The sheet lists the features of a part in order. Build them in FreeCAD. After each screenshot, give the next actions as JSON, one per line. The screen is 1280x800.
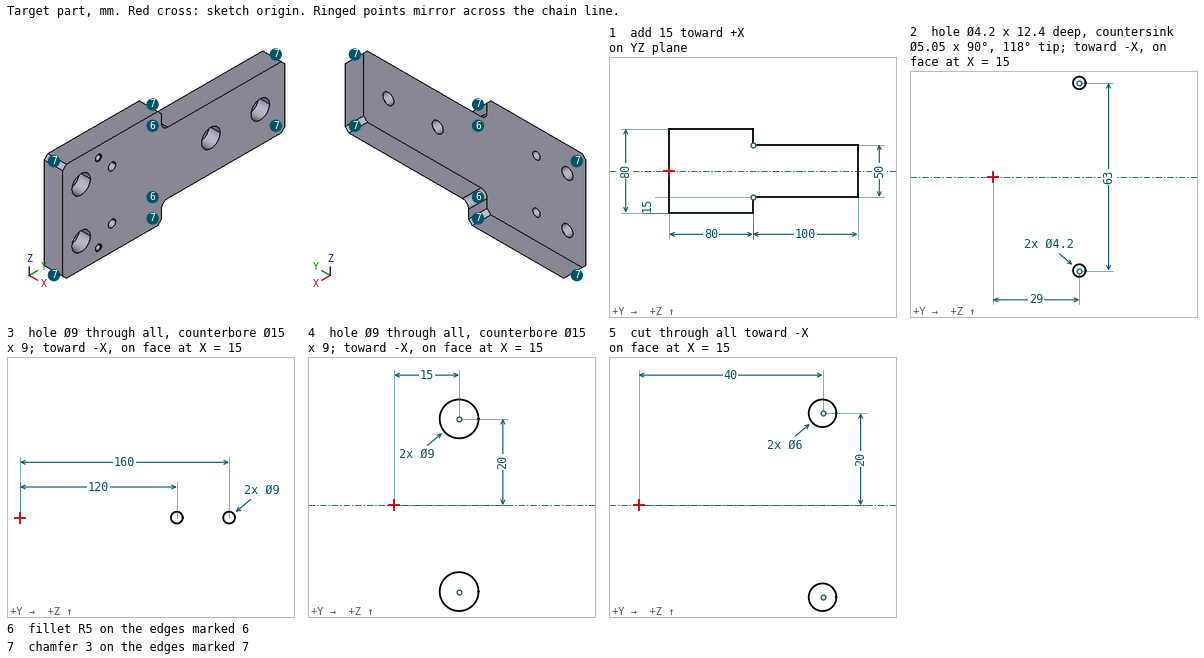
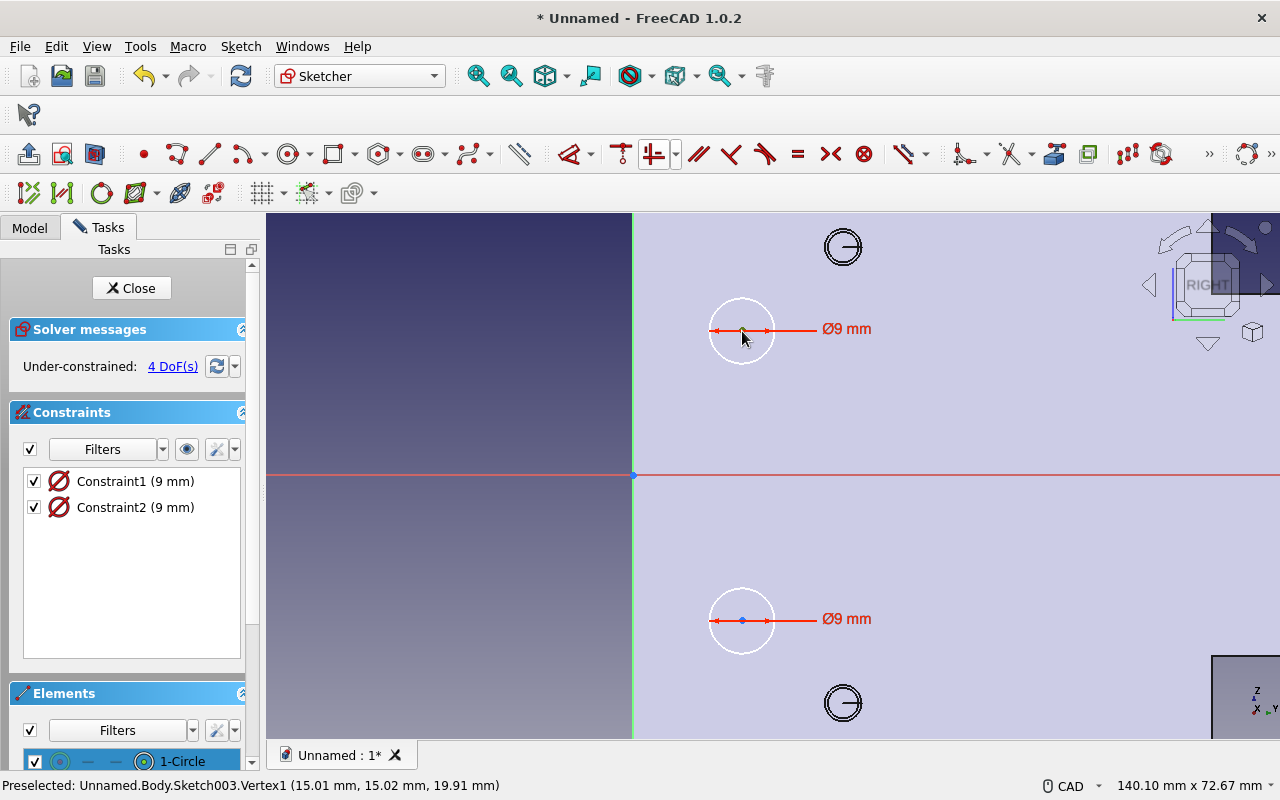
{"action": "left_click", "coordinate": [742, 621]}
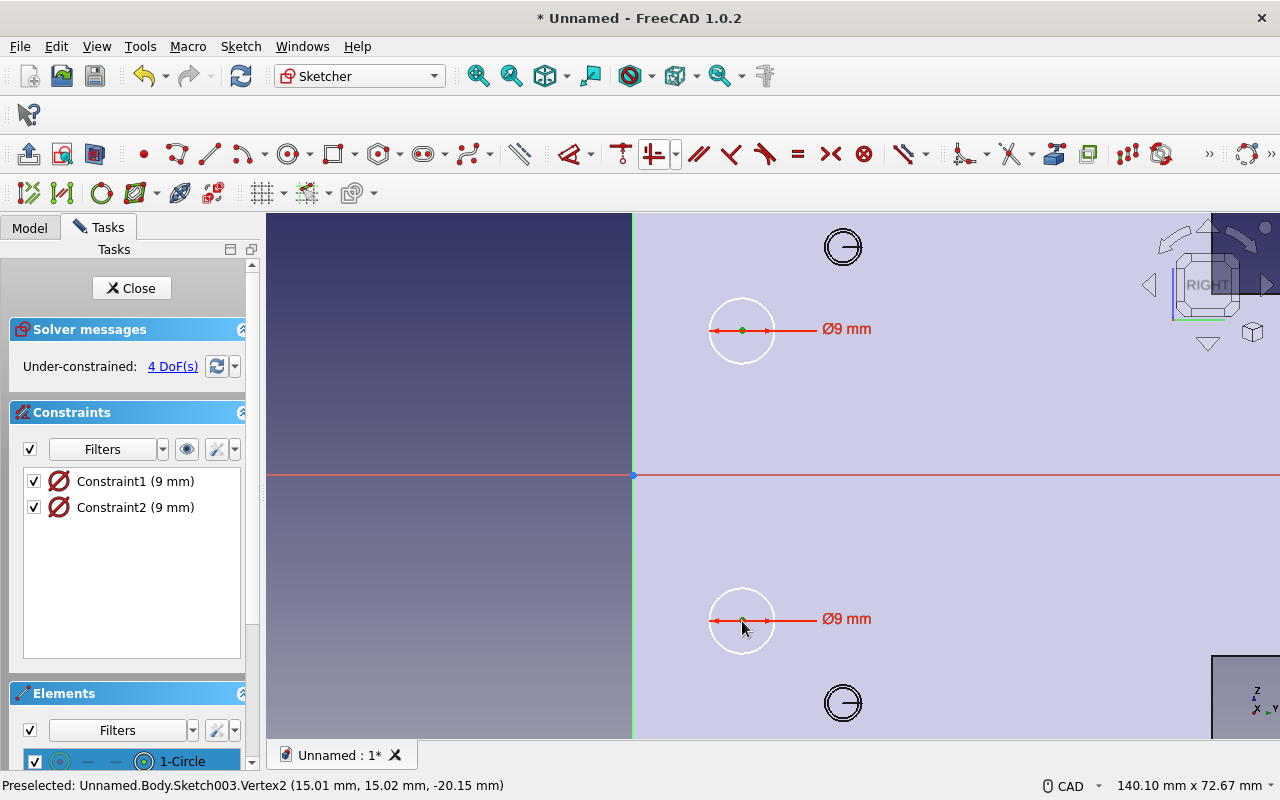
{"action": "left_click", "coordinate": [353, 475]}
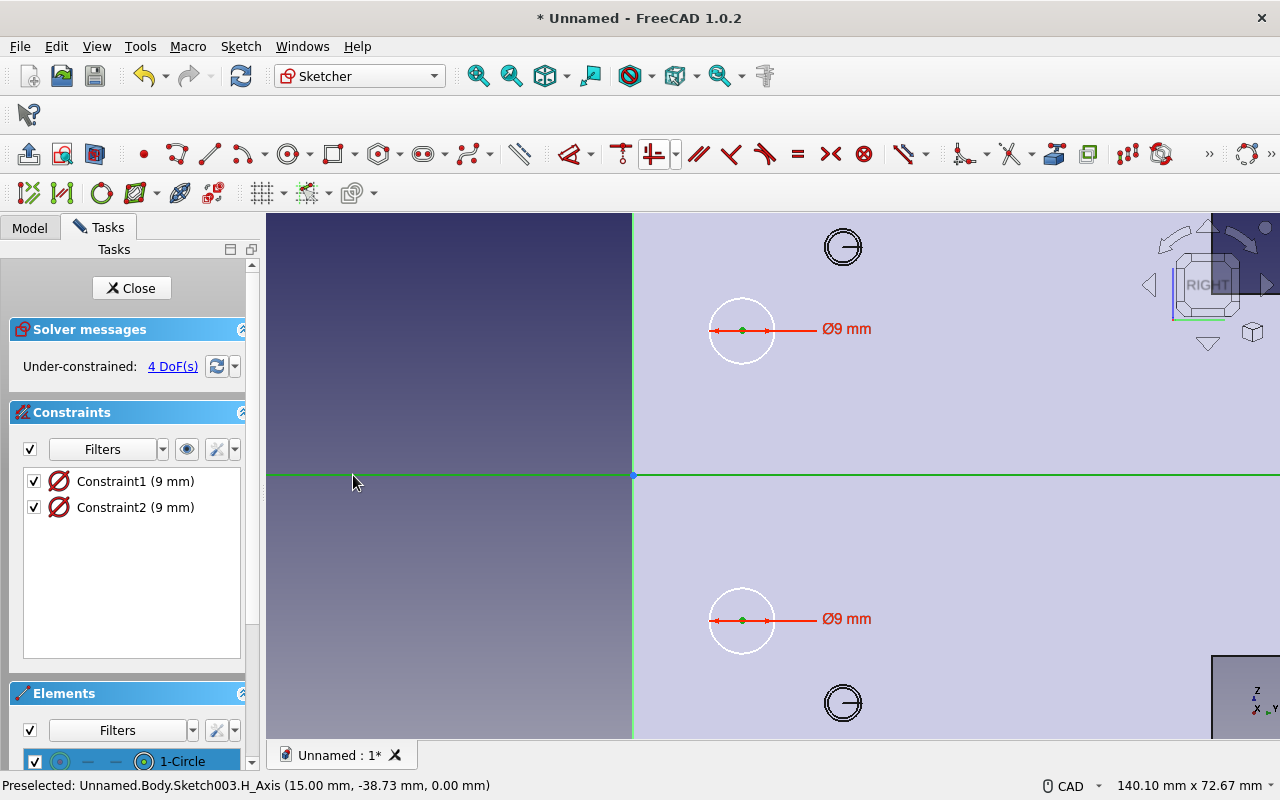
{"action": "left_click", "coordinate": [831, 154]}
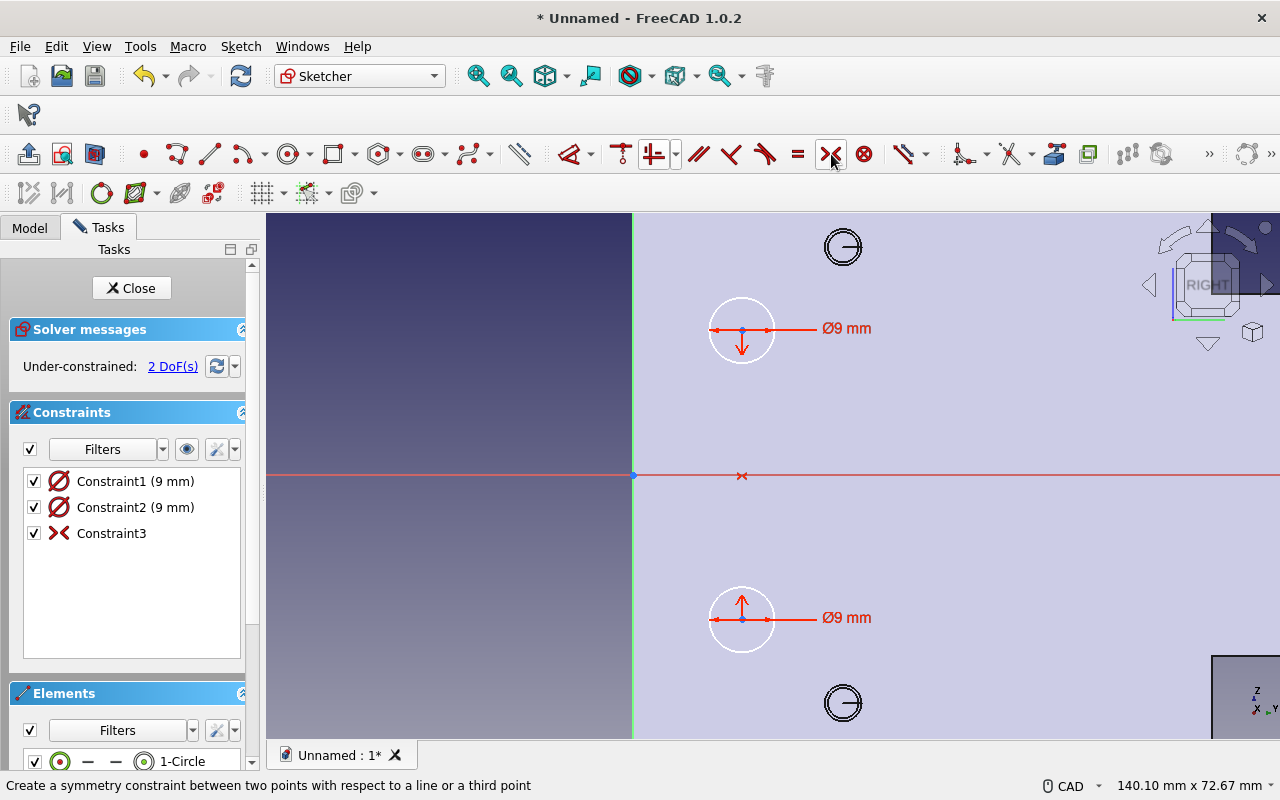
{"action": "left_click", "coordinate": [568, 154]}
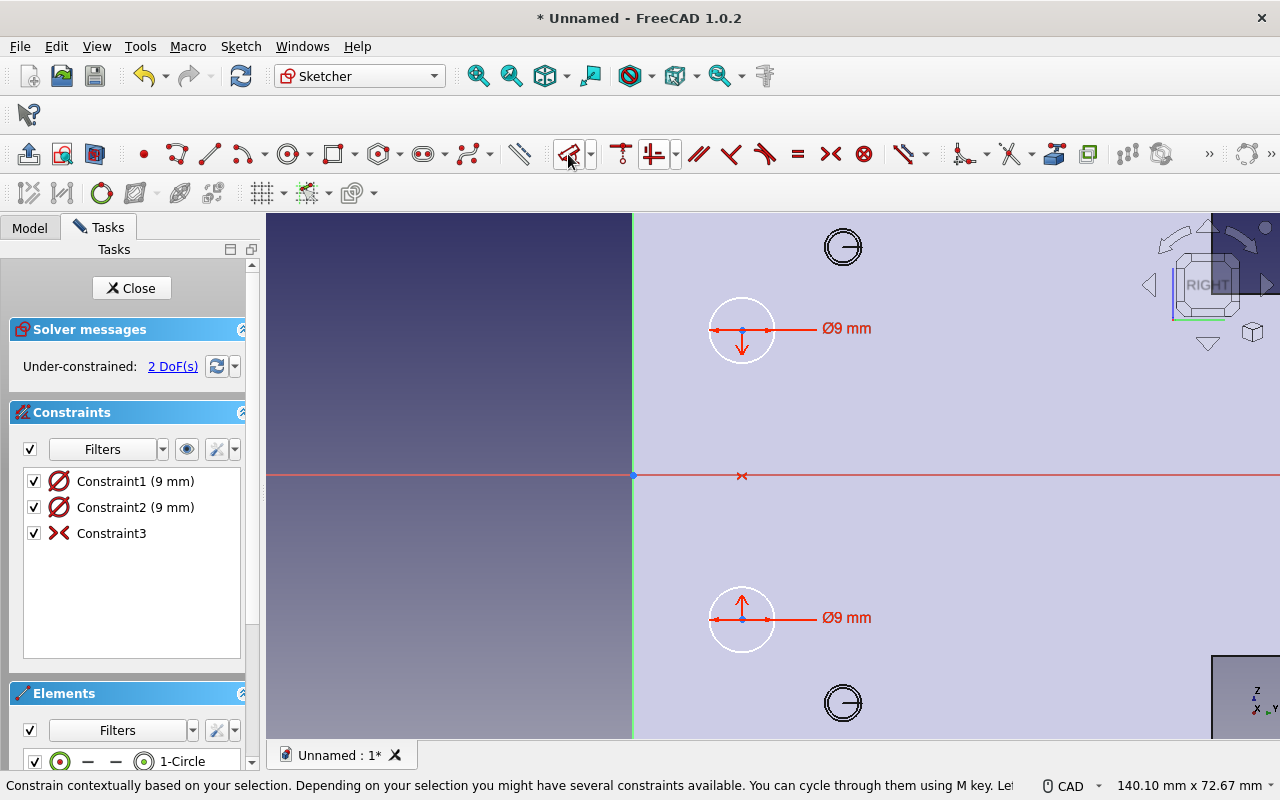
{"action": "left_click", "coordinate": [742, 330]}
{"action": "left_click", "coordinate": [688, 296]}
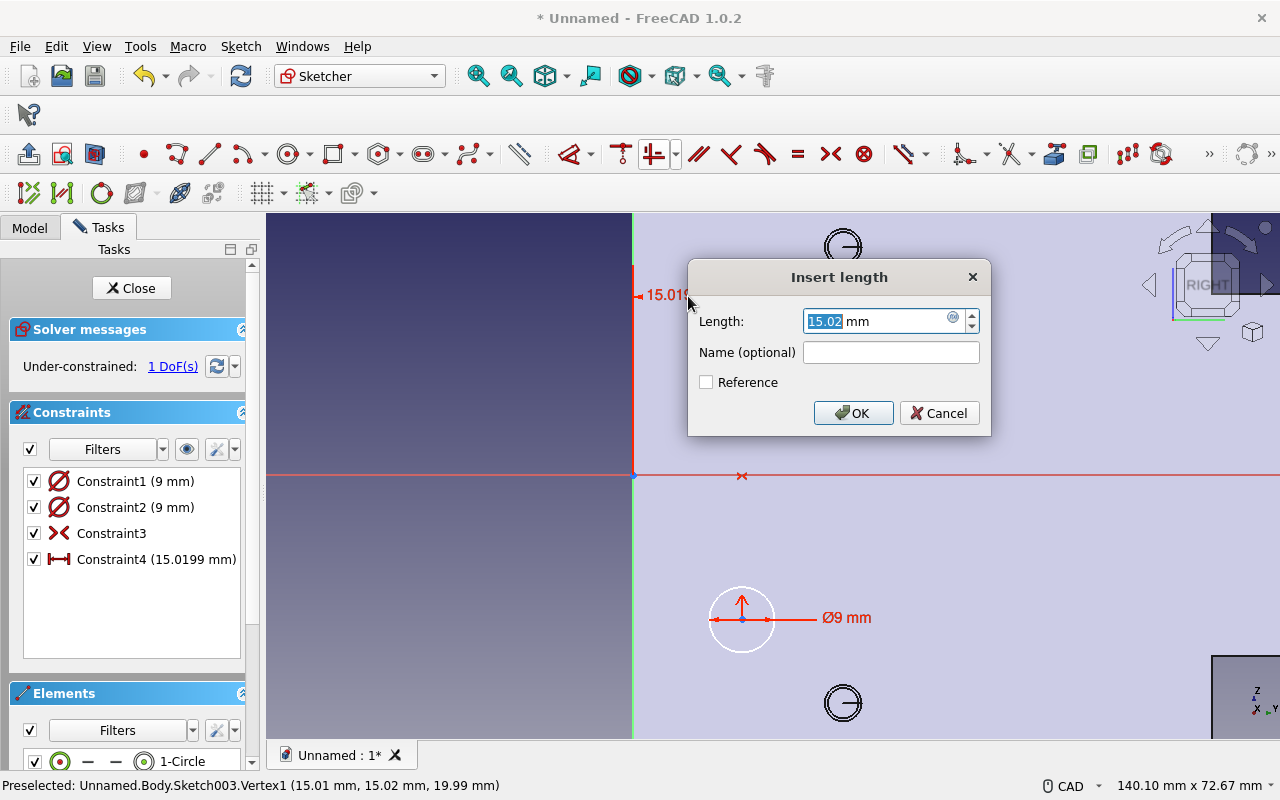
{"action": "type", "text": "15"}
{"action": "key", "text": "Return"}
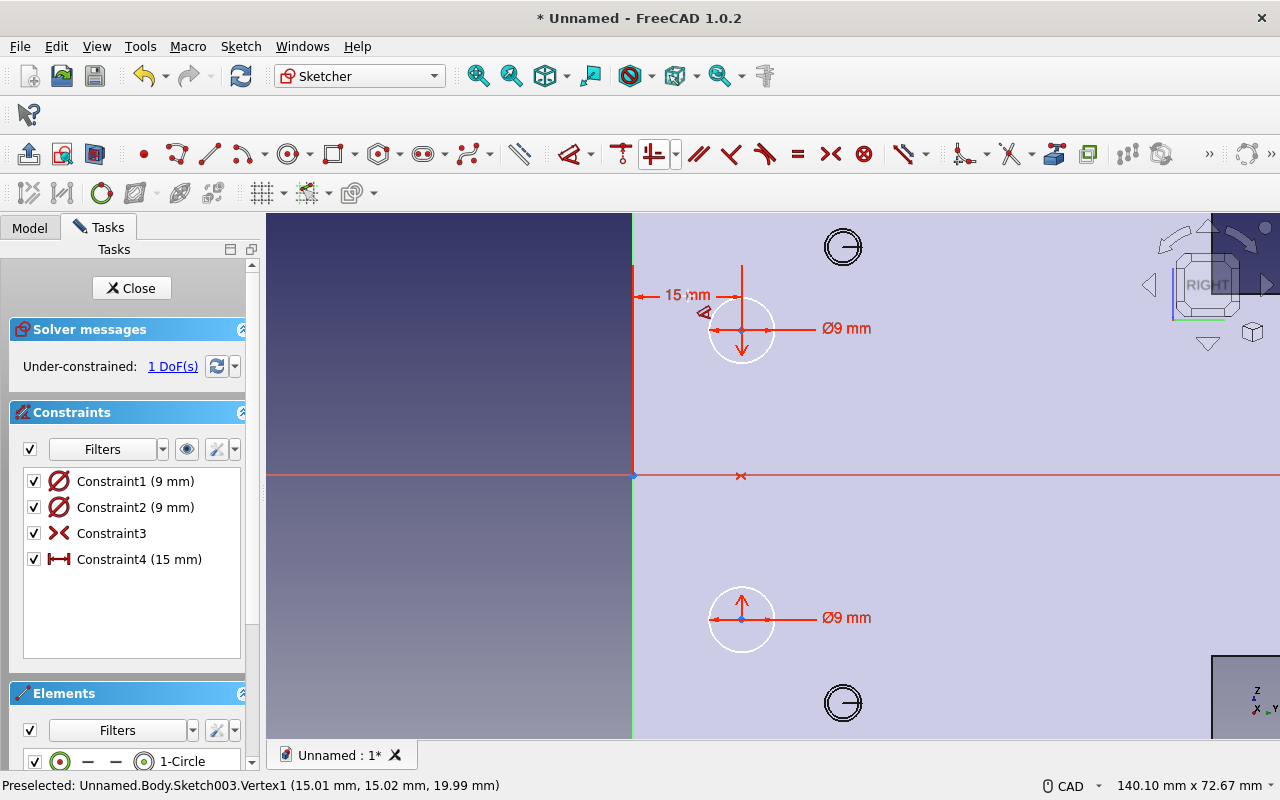
{"action": "left_click", "coordinate": [742, 330]}
{"action": "left_click", "coordinate": [599, 403]}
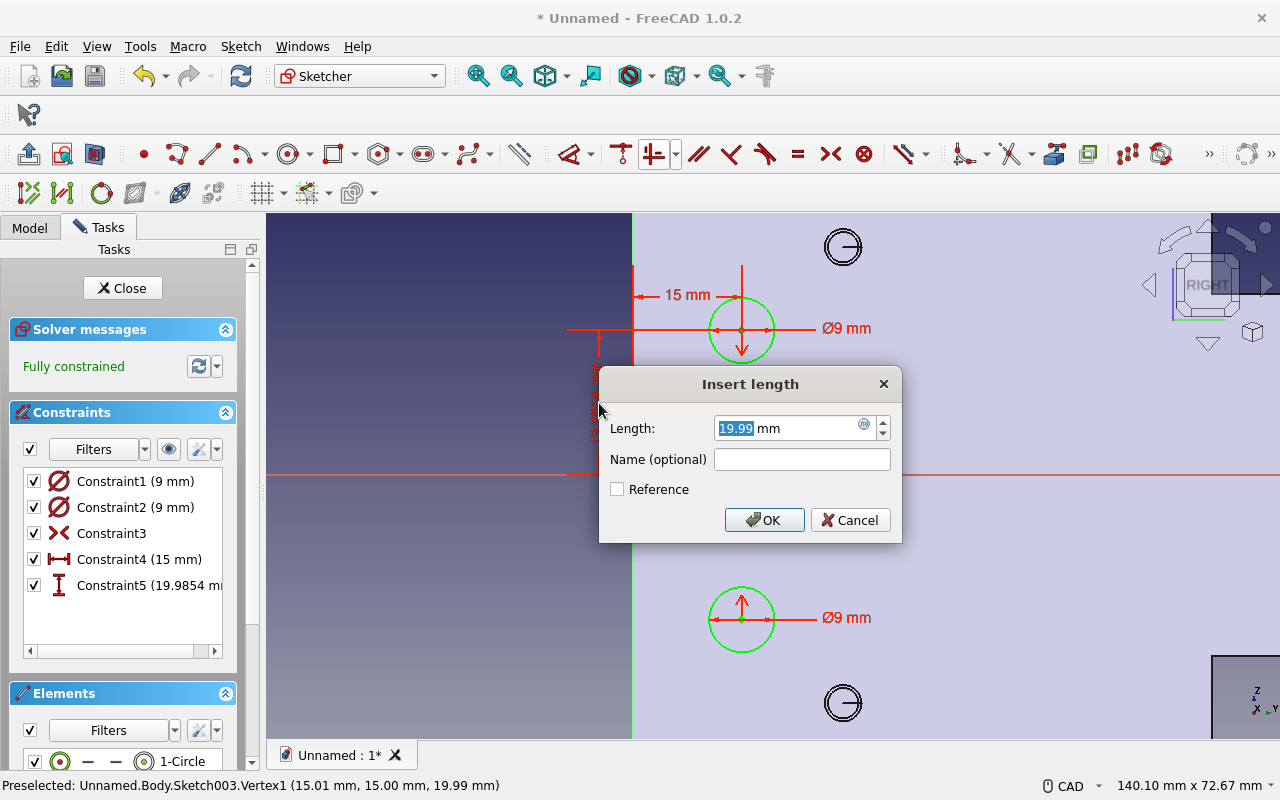
{"action": "type", "text": "20"}
{"action": "key", "text": "Return"}
{"action": "key", "text": "Escape"}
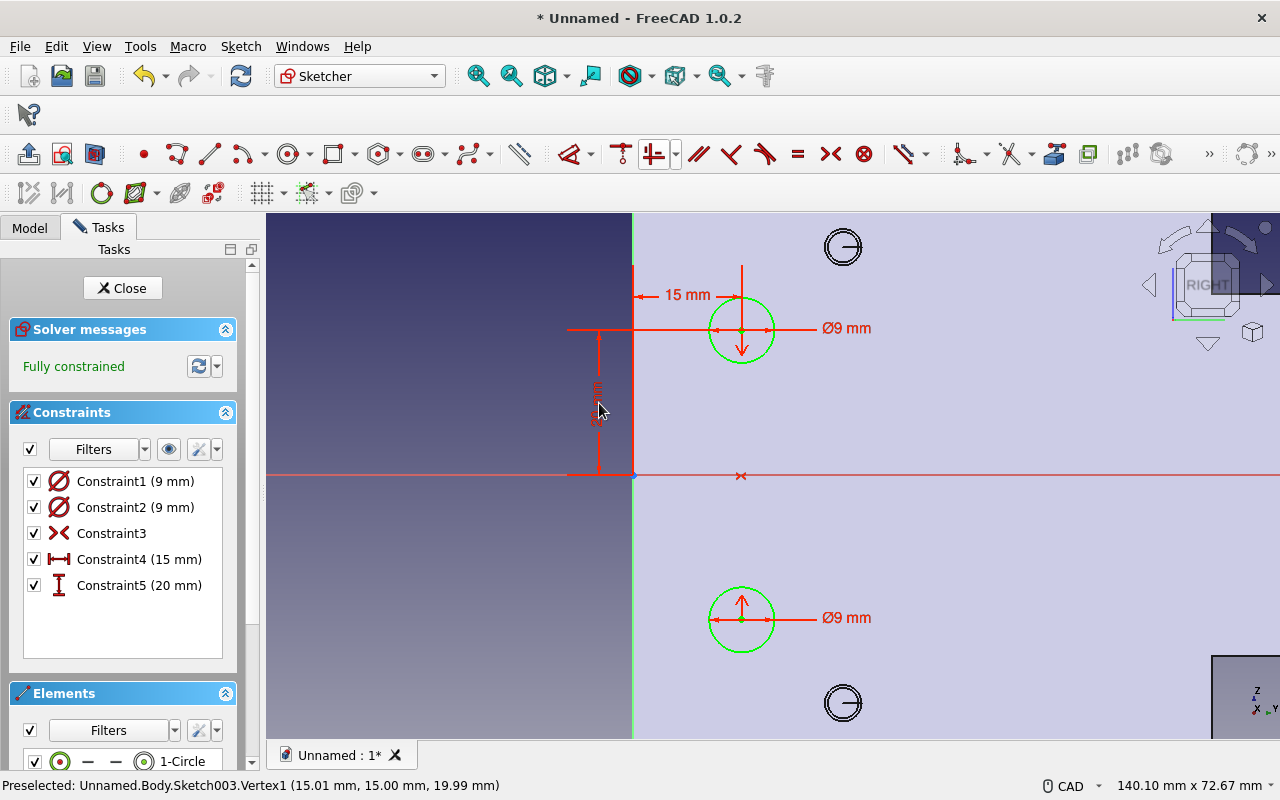
{"action": "left_click", "coordinate": [123, 288]}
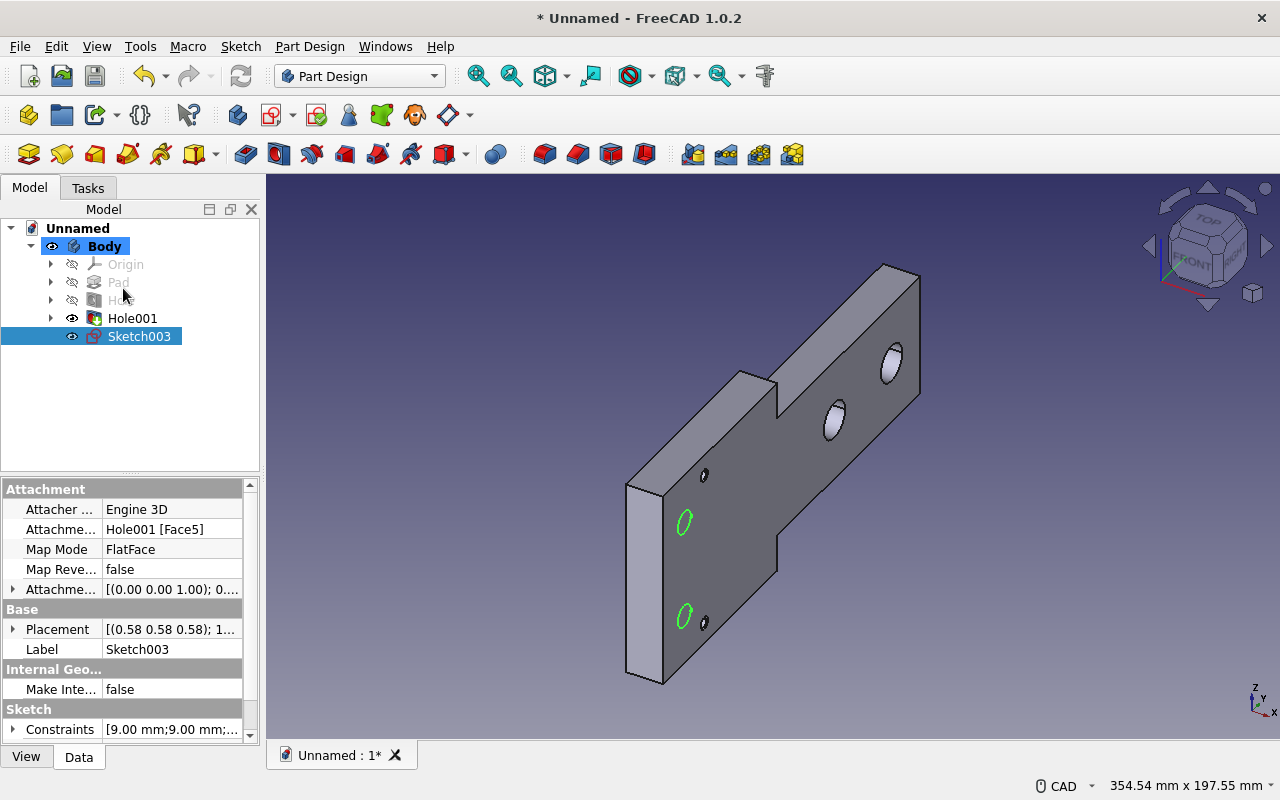
{"action": "left_click", "coordinate": [279, 154]}